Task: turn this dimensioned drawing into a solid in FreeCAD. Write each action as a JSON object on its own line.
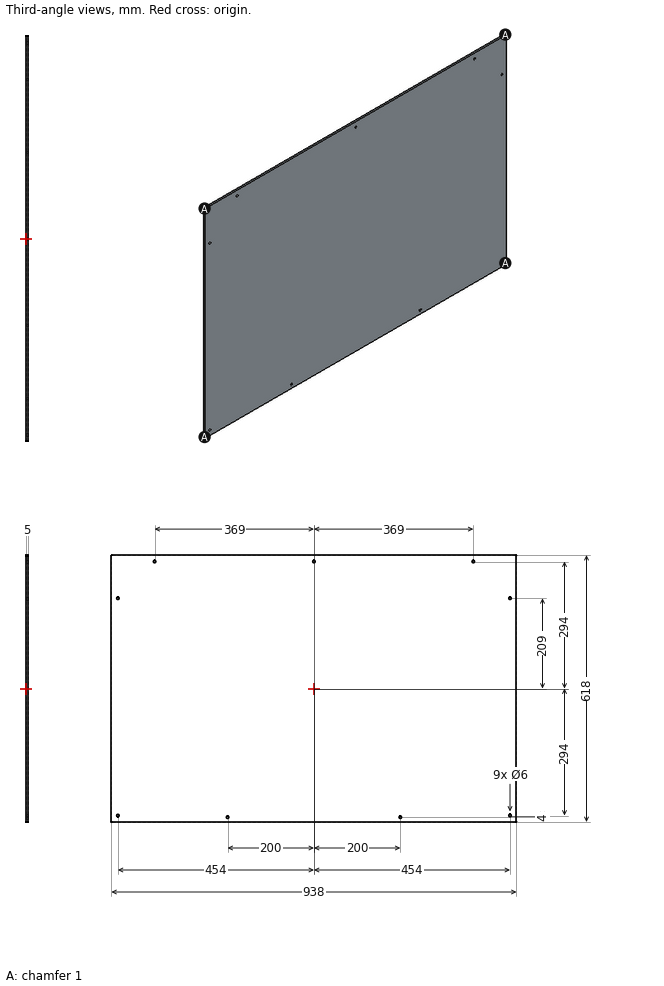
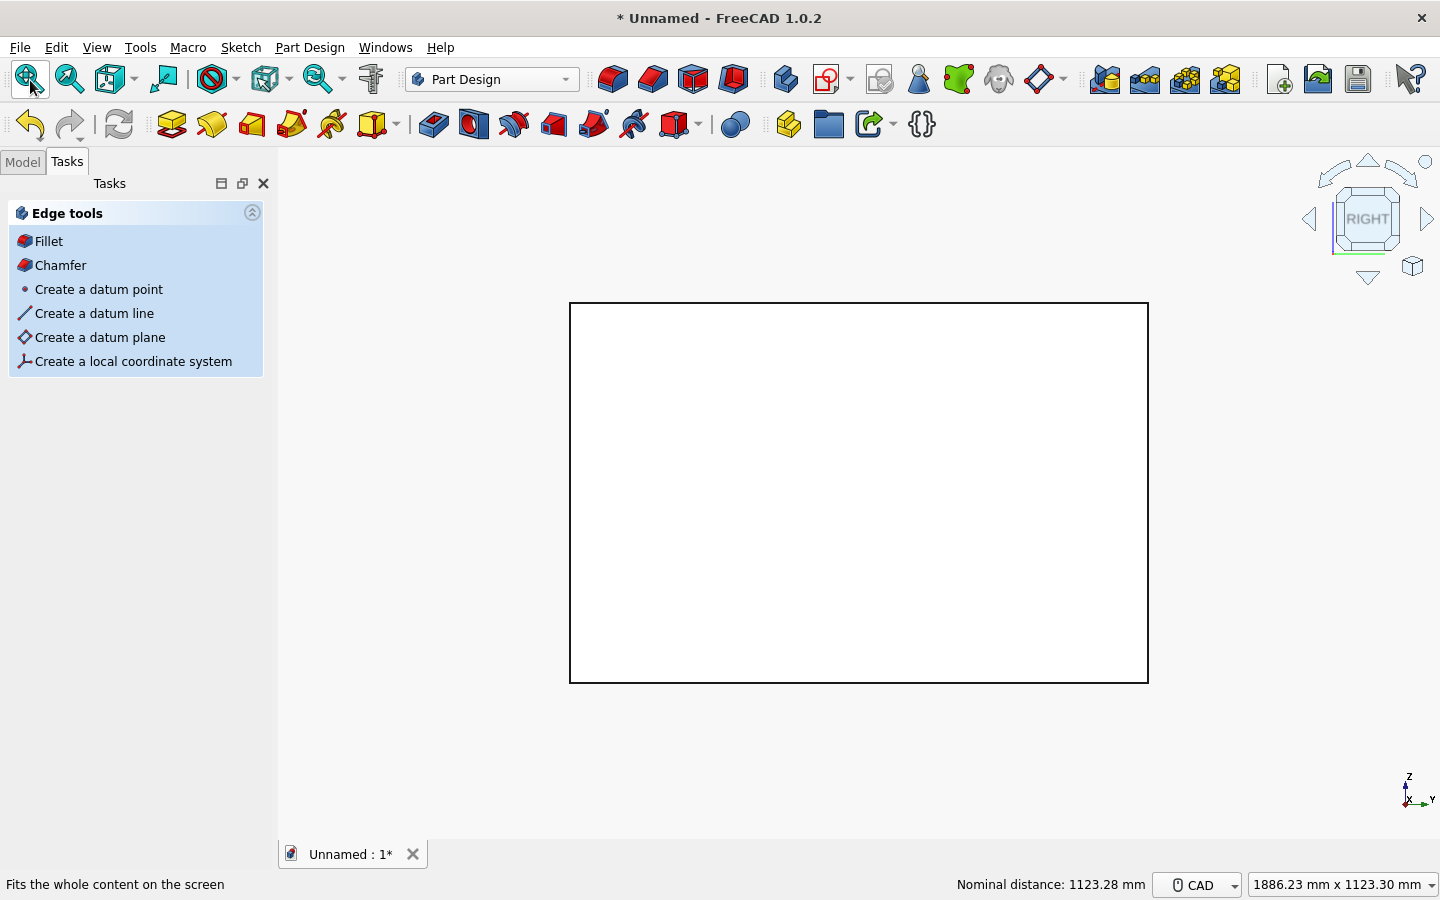
{"action": "scroll", "coordinate": [1148, 682], "scroll_direction": "up", "scroll_amount": 13}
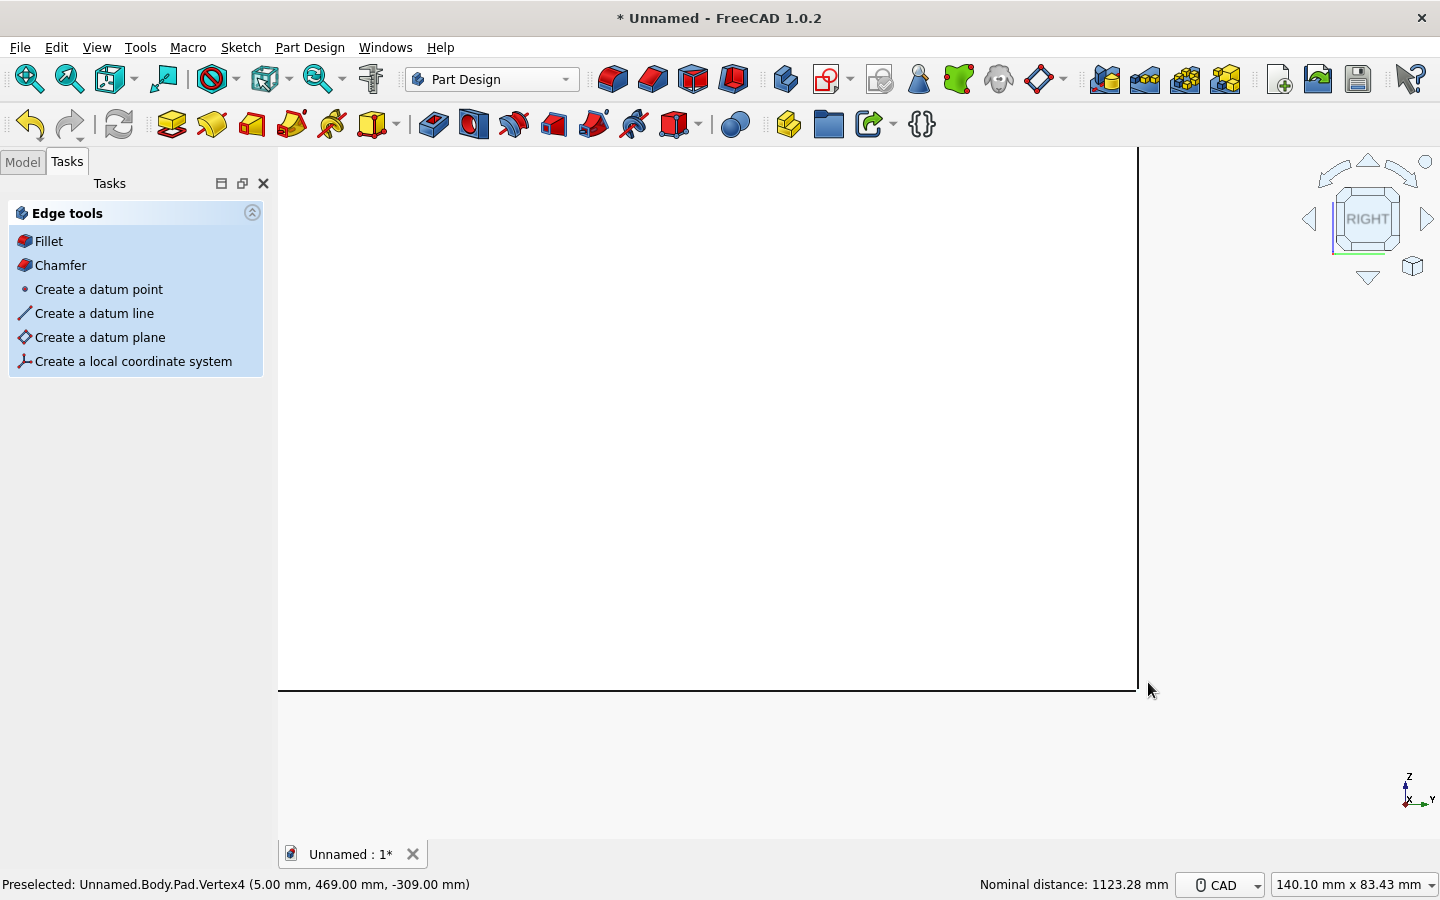
{"action": "left_click", "coordinate": [30, 80]}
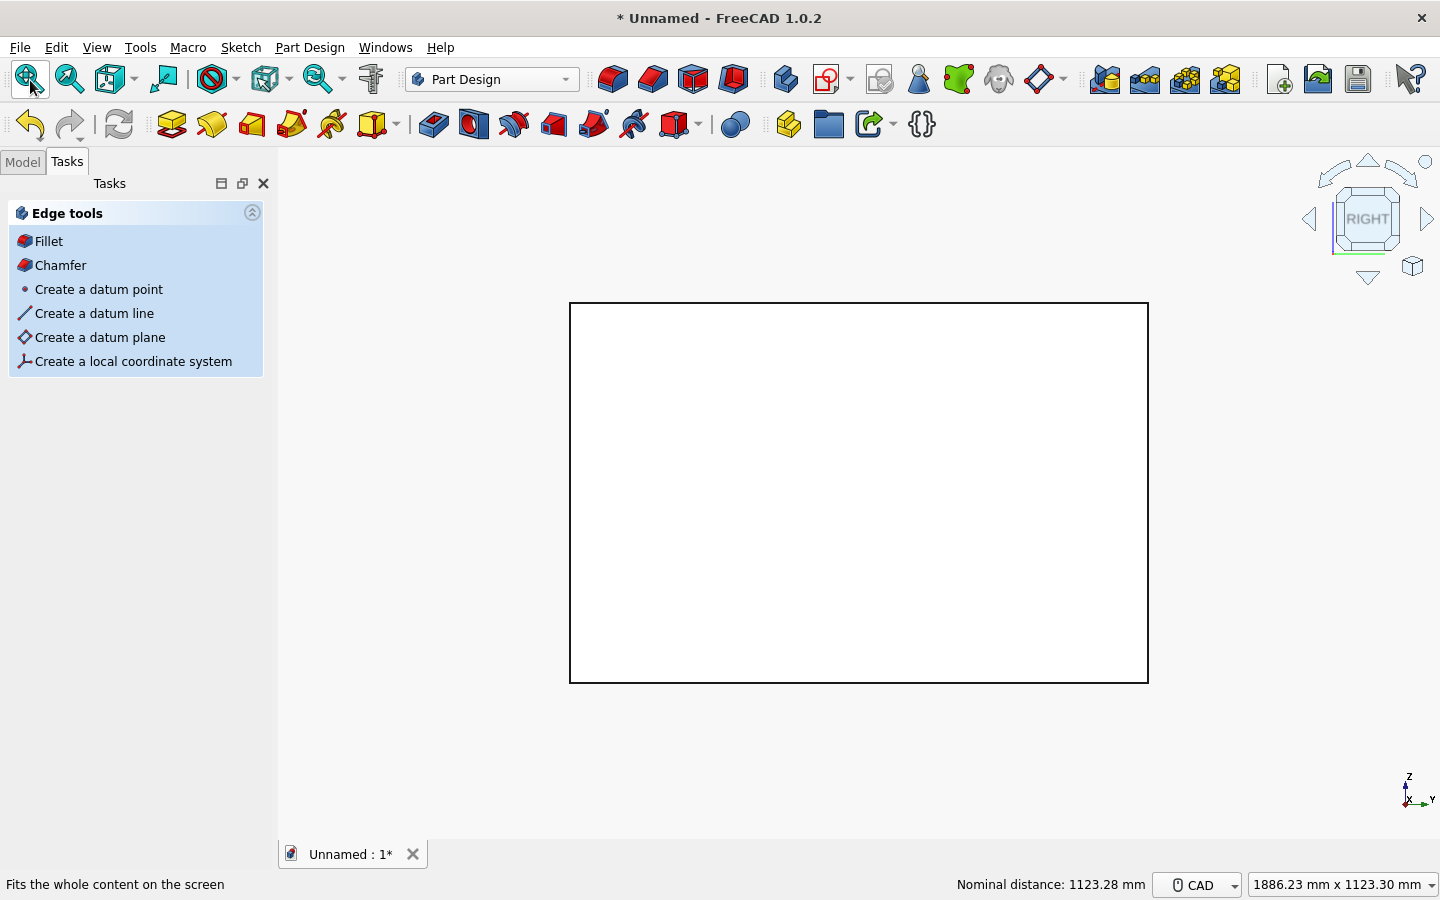
{"action": "key", "text": "5"}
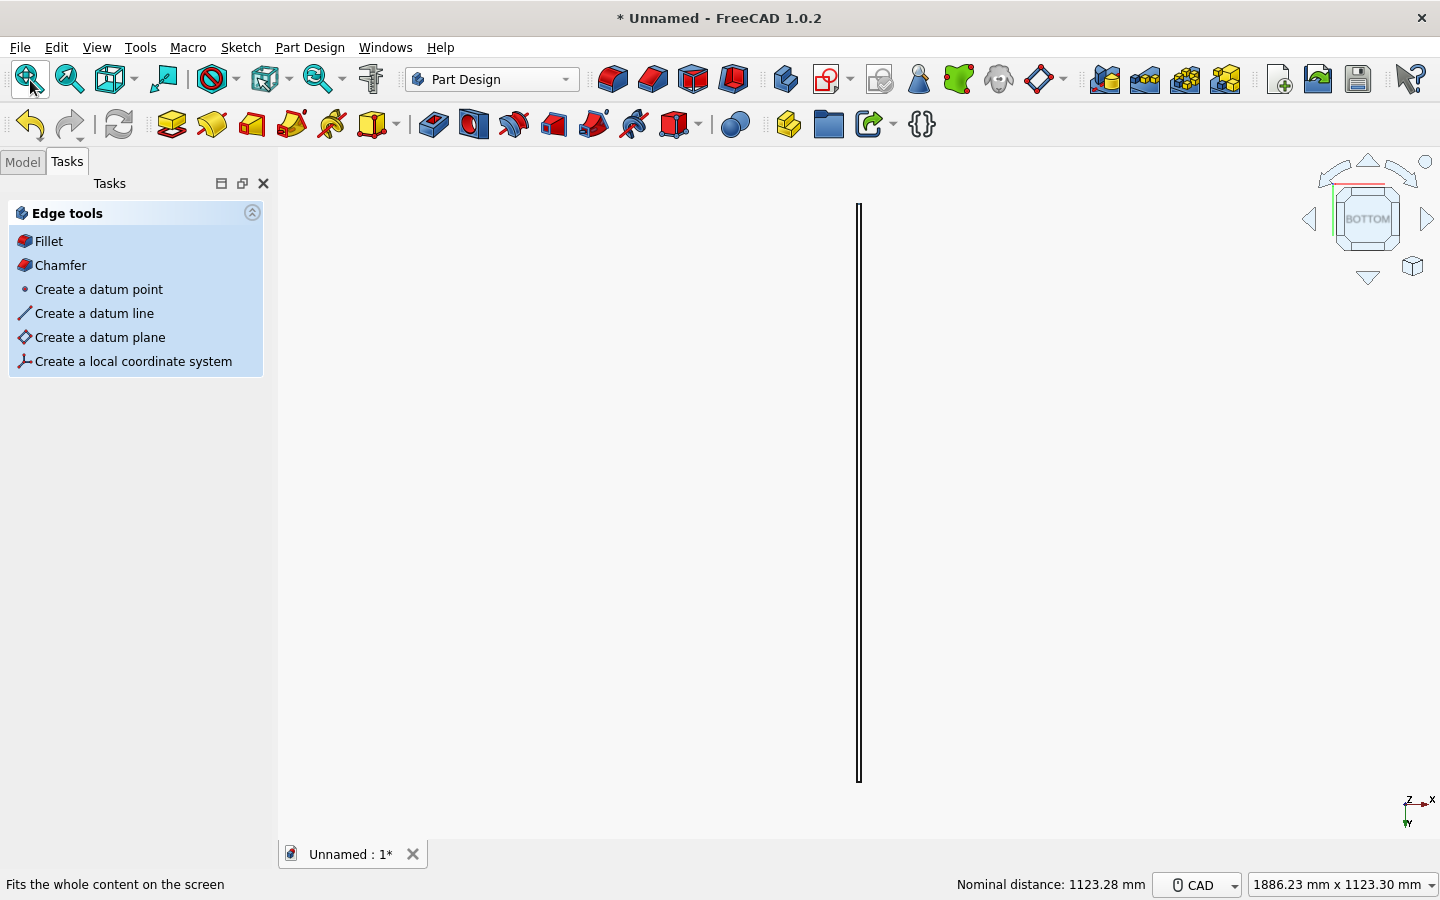
{"action": "scroll", "coordinate": [859, 781], "scroll_direction": "up", "scroll_amount": 13}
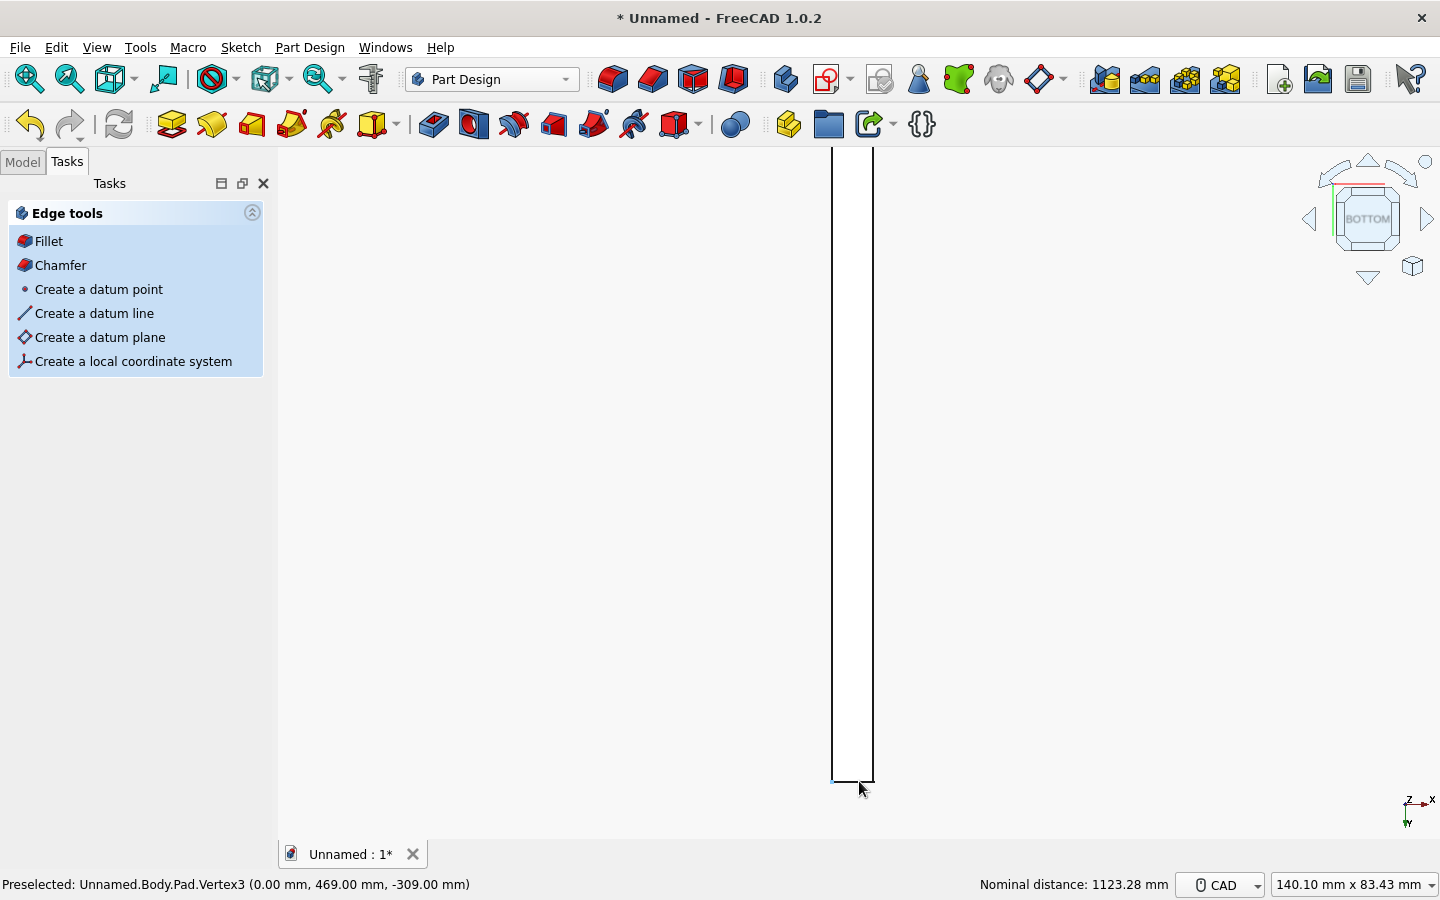
{"action": "left_click", "coordinate": [853, 781], "text": "ctrl"}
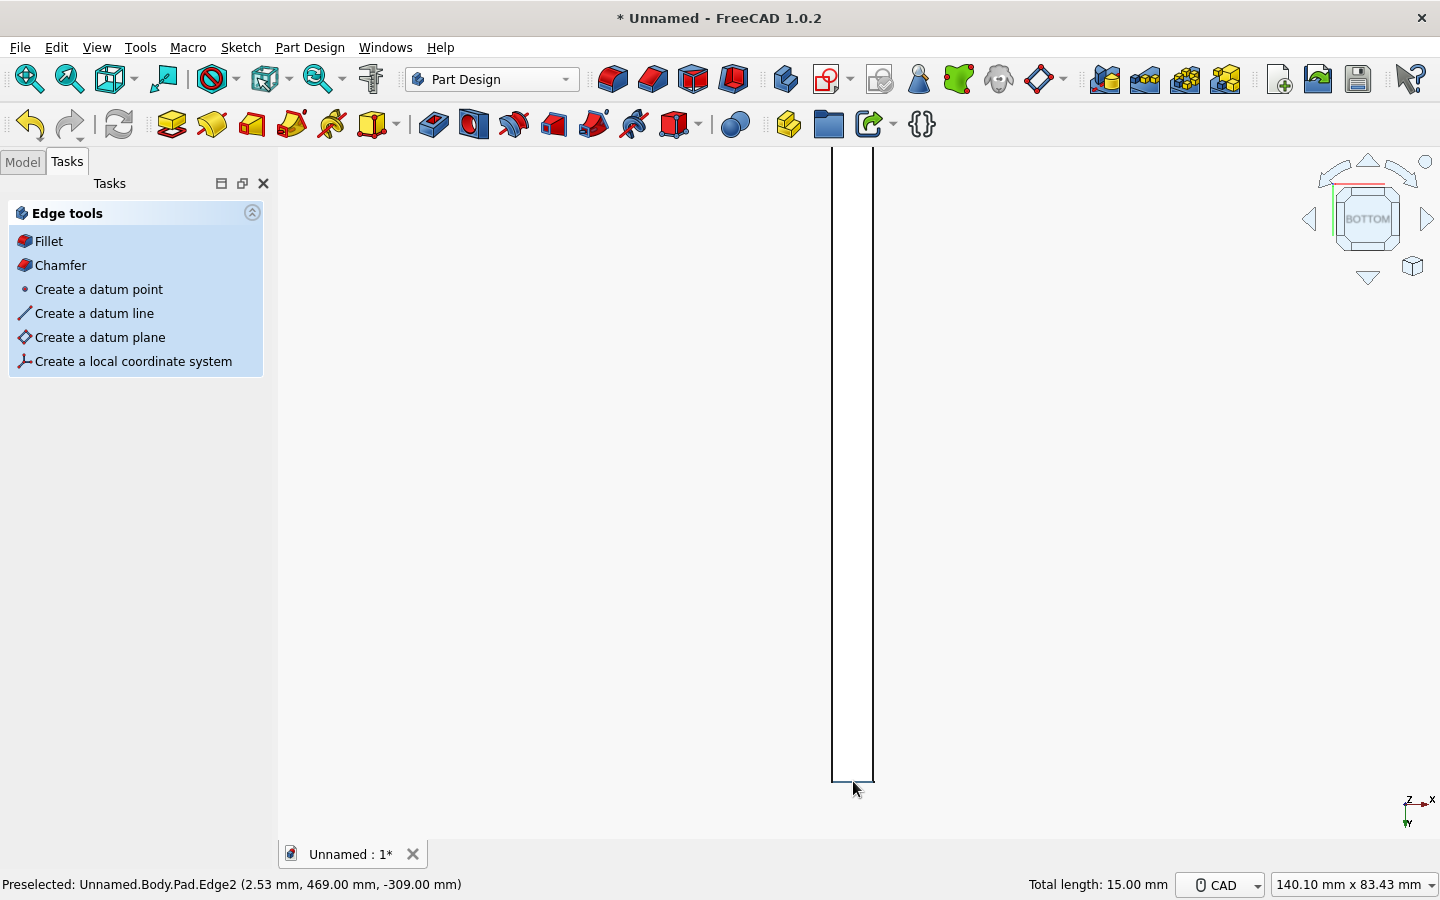
{"action": "left_click", "coordinate": [30, 80]}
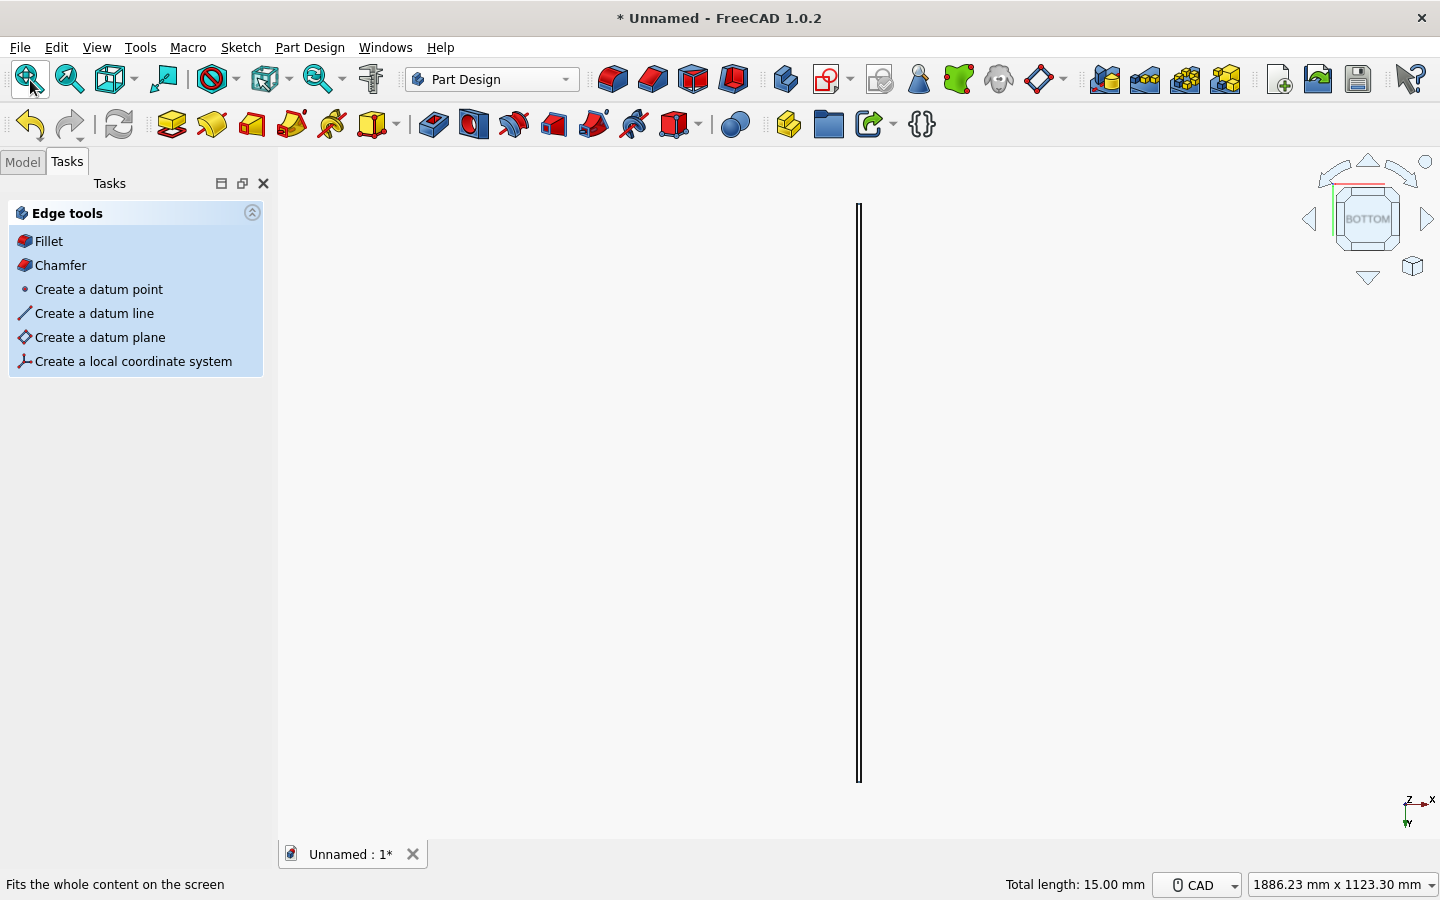
{"action": "key", "text": "4"}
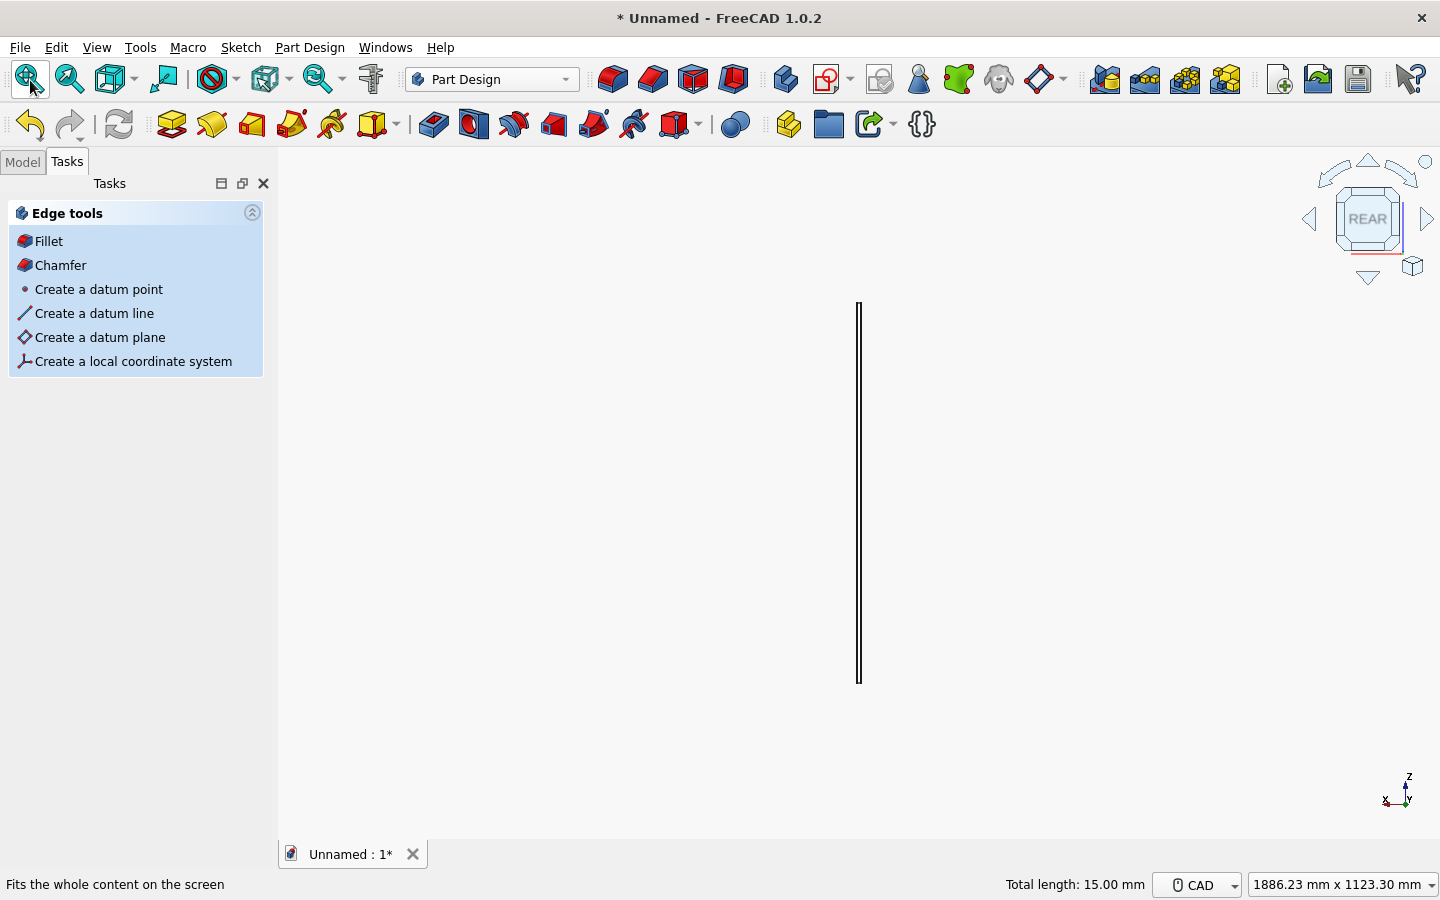
{"action": "scroll", "coordinate": [859, 302], "scroll_direction": "up", "scroll_amount": 13}